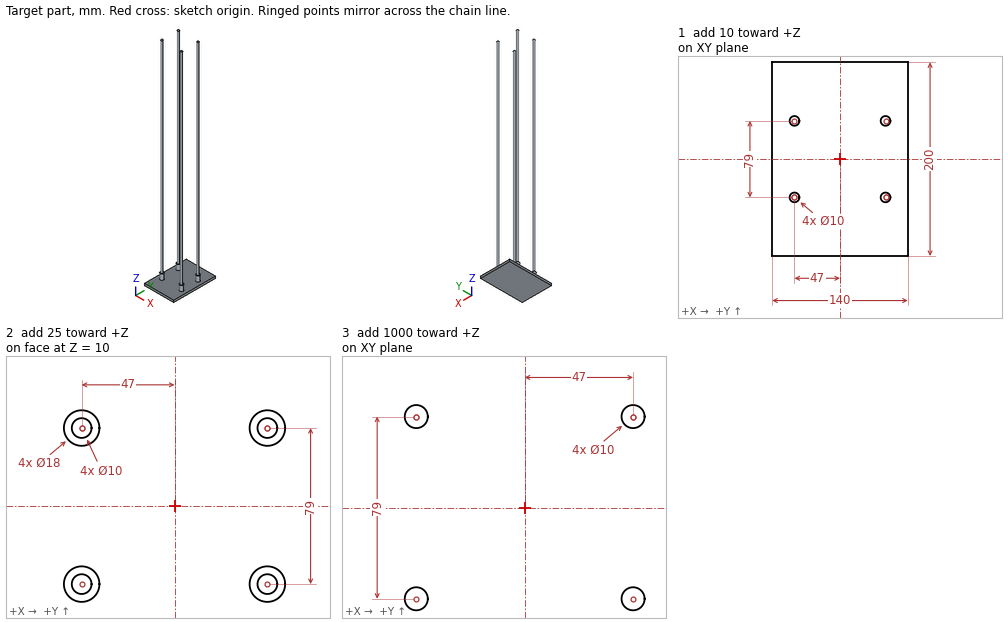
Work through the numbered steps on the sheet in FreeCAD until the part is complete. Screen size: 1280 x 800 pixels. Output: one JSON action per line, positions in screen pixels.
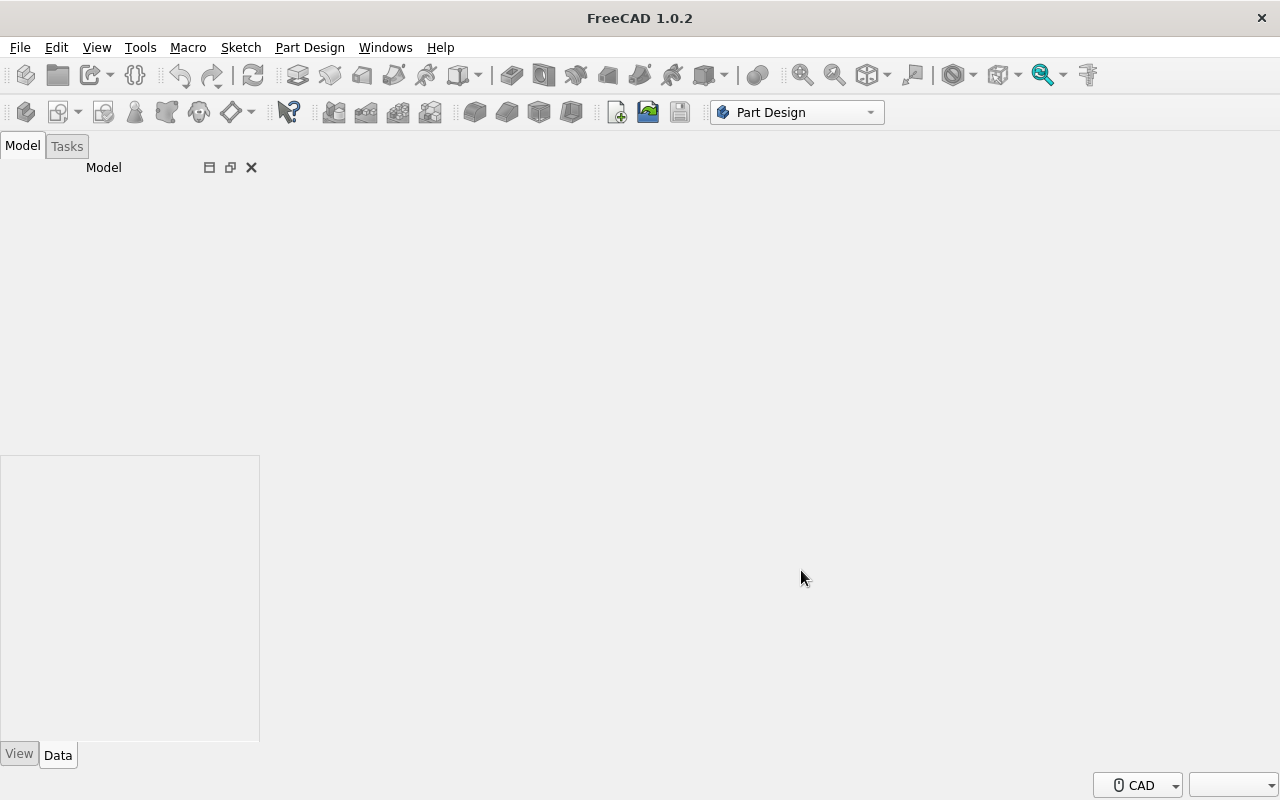
{"action": "left_click", "coordinate": [616, 112]}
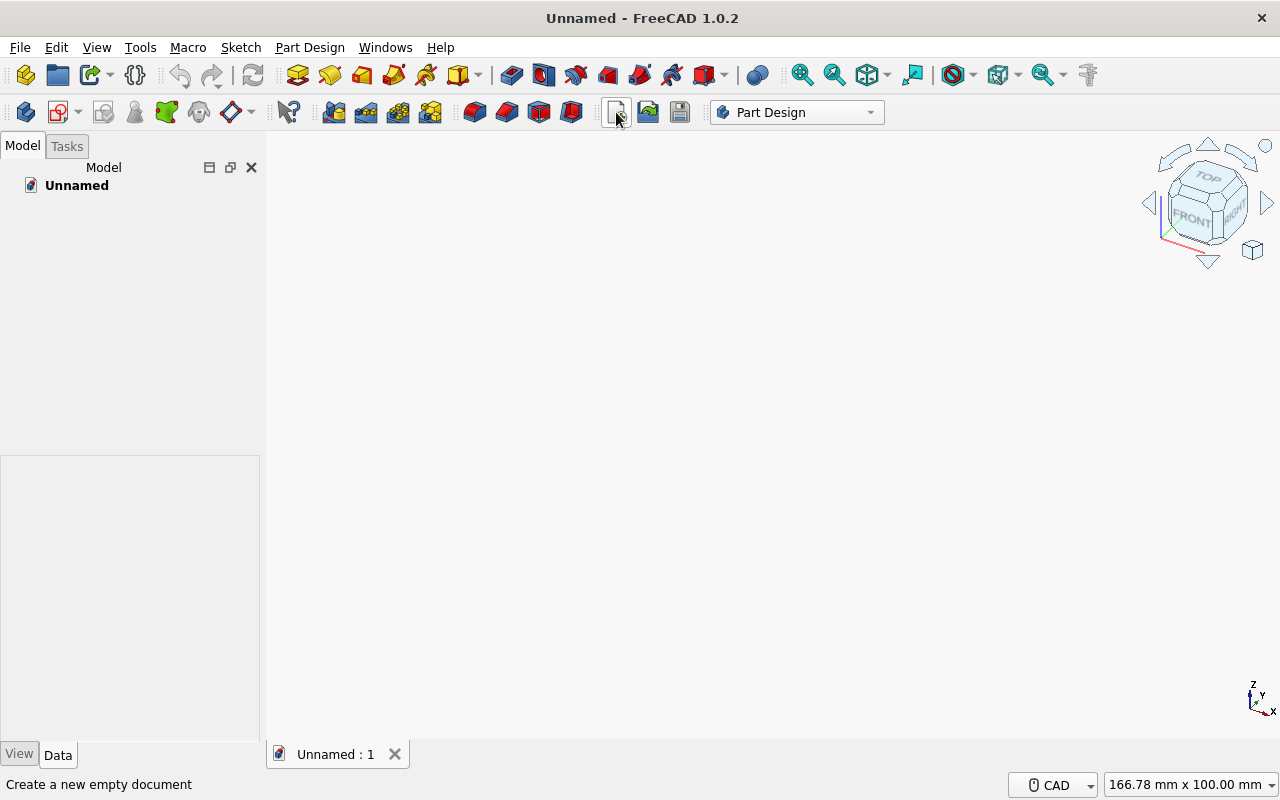
{"action": "left_click", "coordinate": [58, 112]}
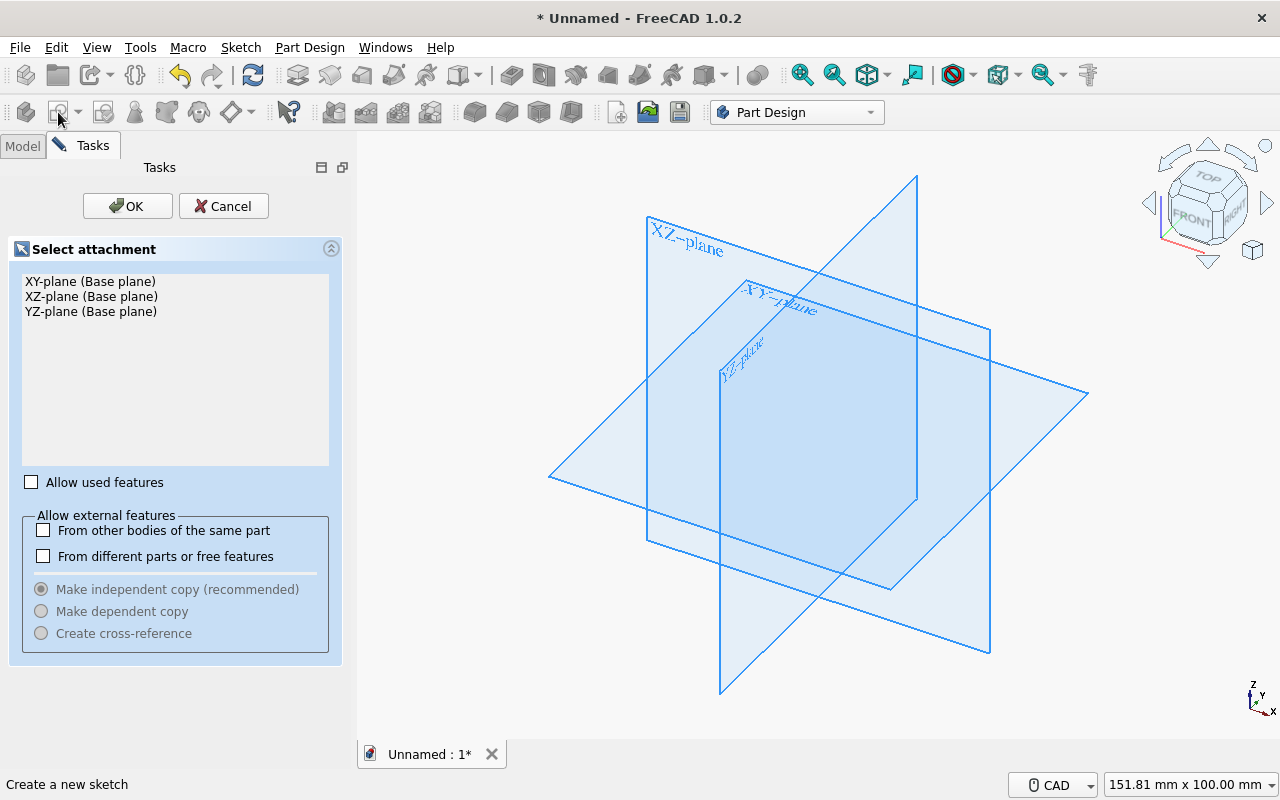
{"action": "left_click", "coordinate": [82, 282]}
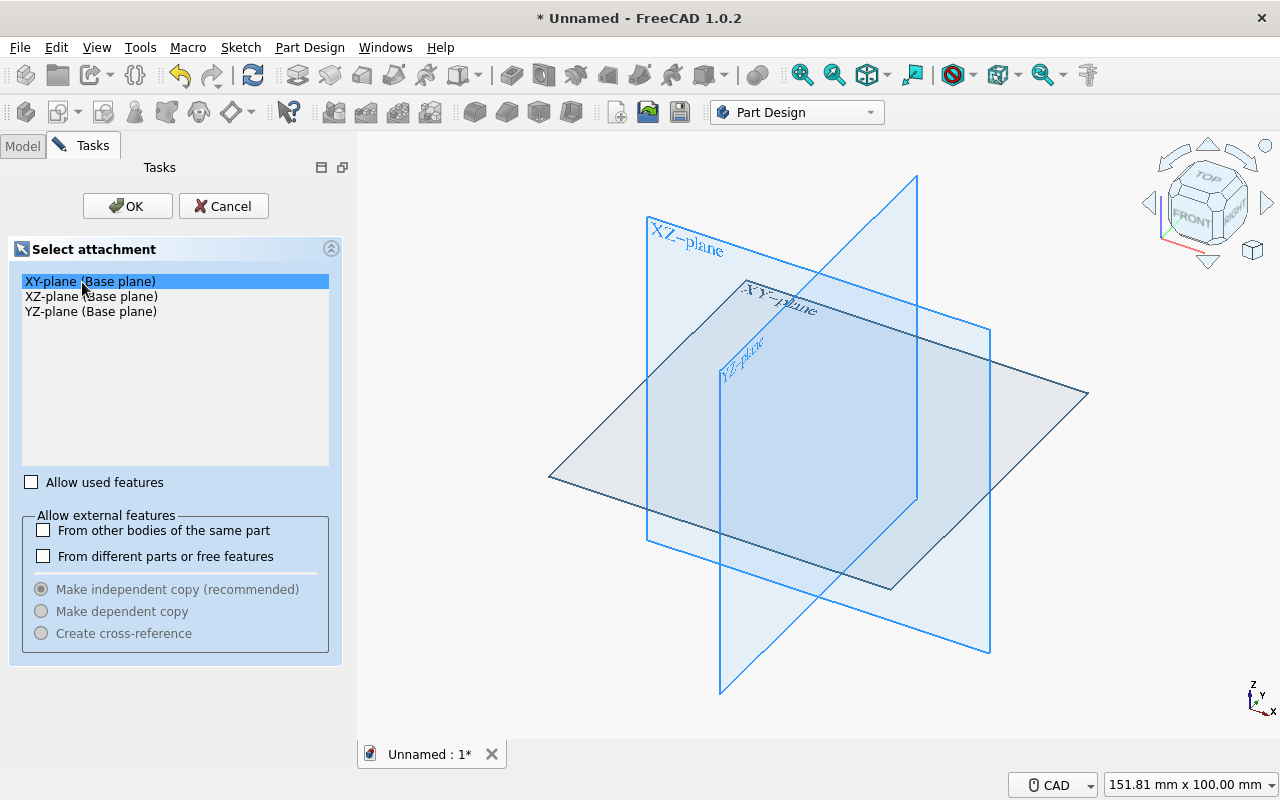
{"action": "left_click", "coordinate": [128, 206]}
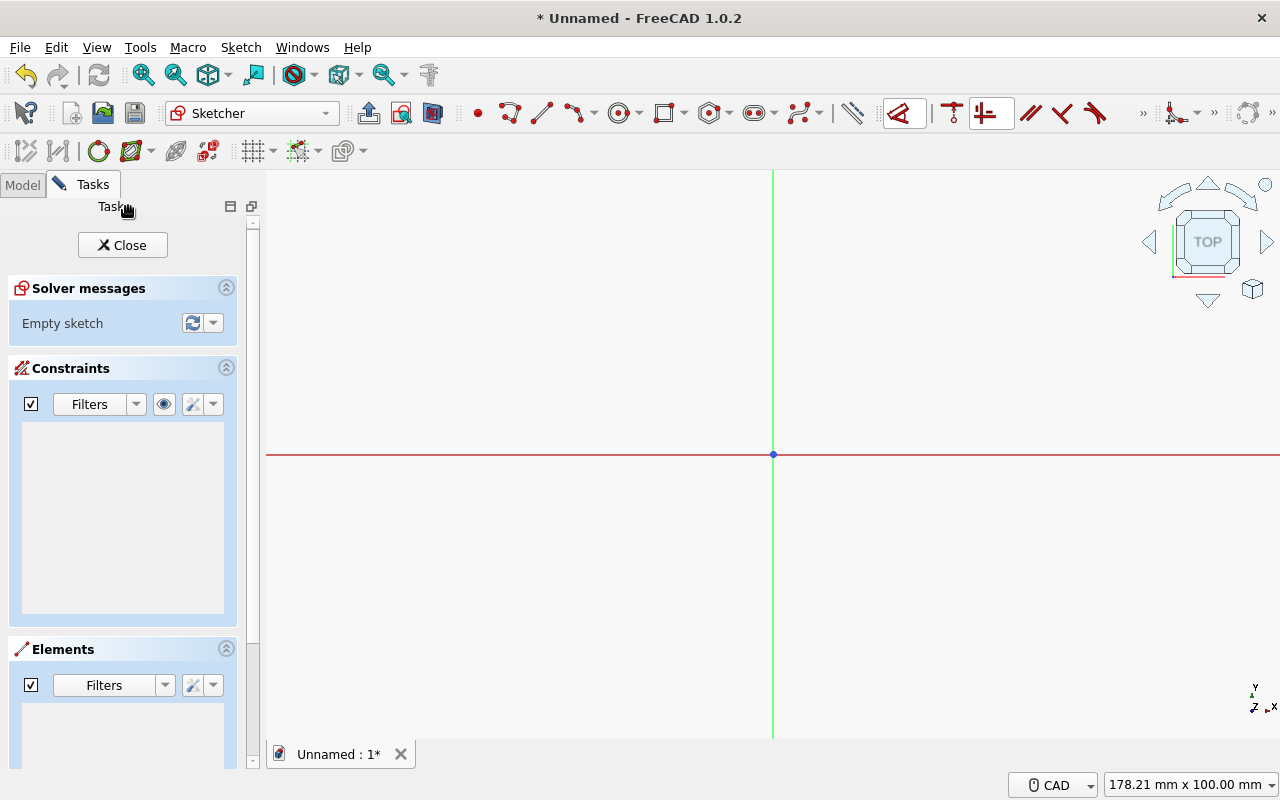
{"action": "scroll", "coordinate": [675, 454], "scroll_direction": "down", "scroll_amount": 6}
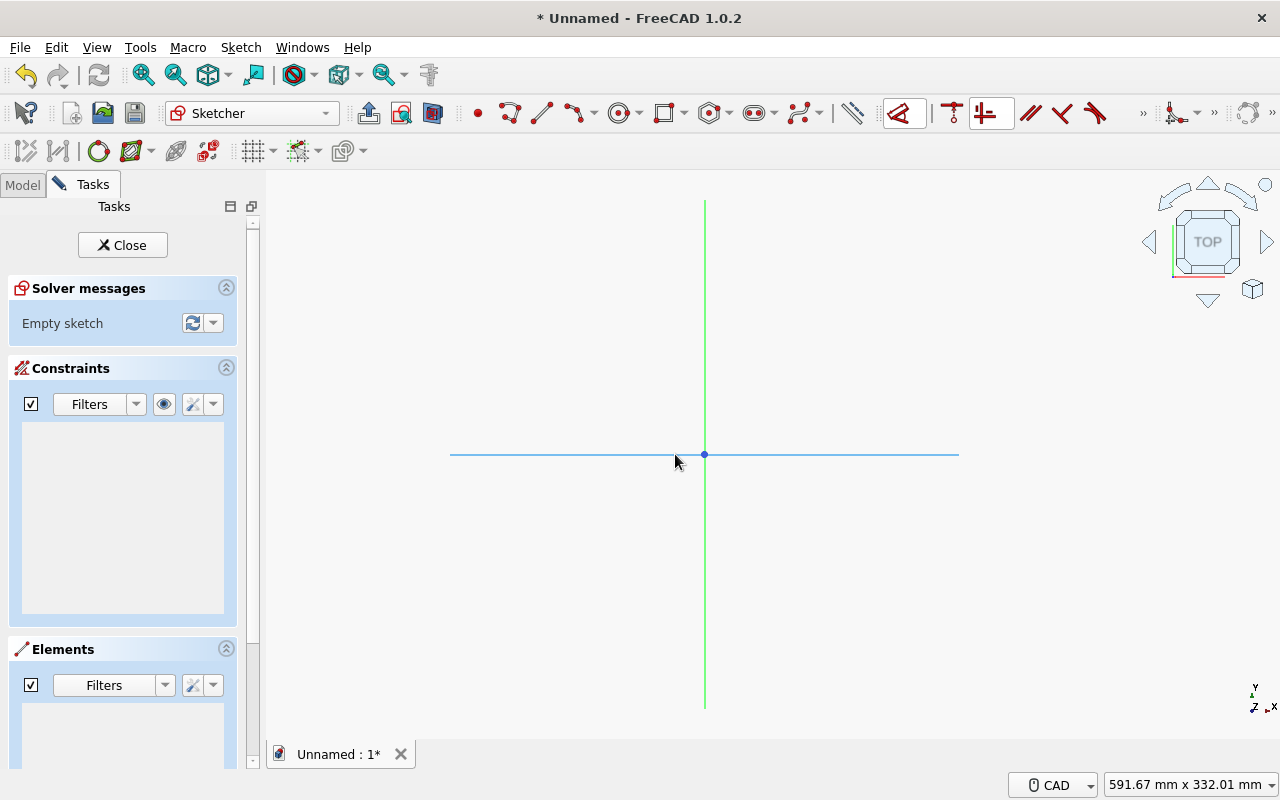
{"action": "left_click", "coordinate": [686, 114]}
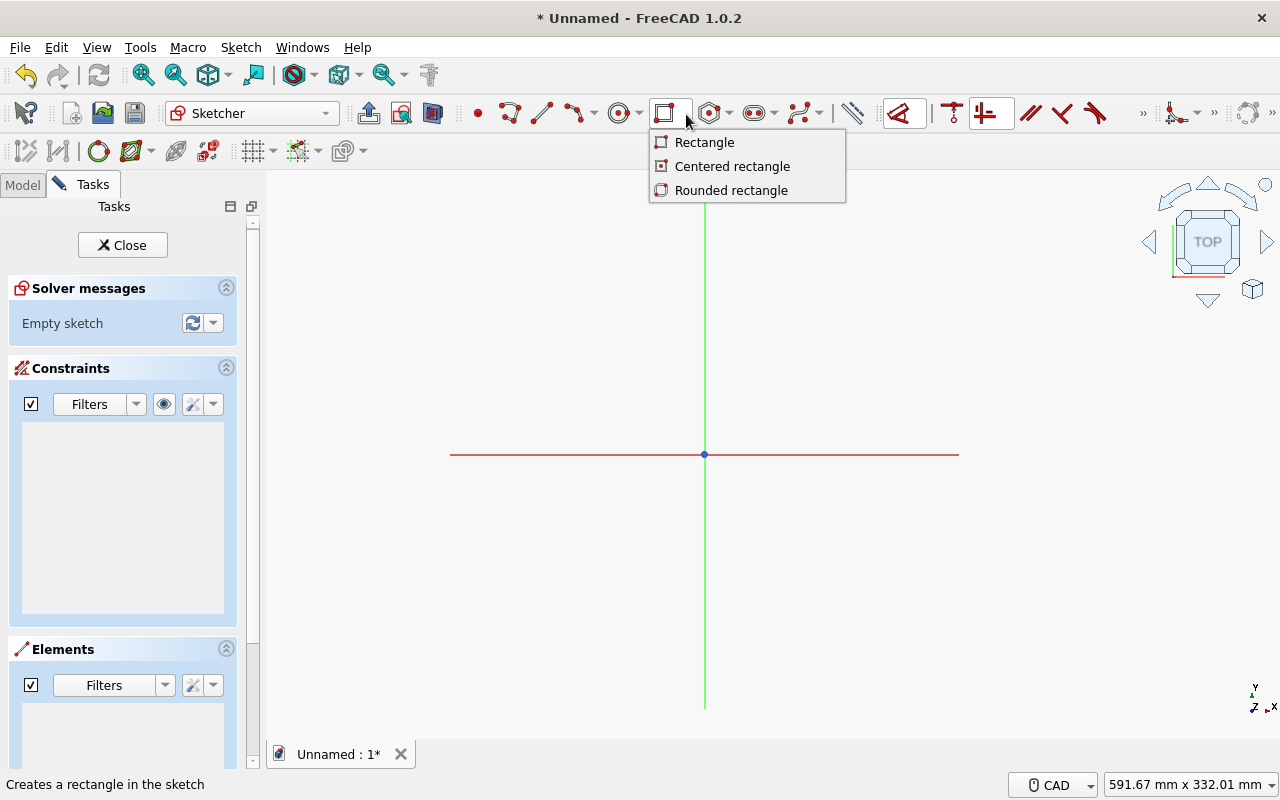
{"action": "left_click", "coordinate": [748, 166]}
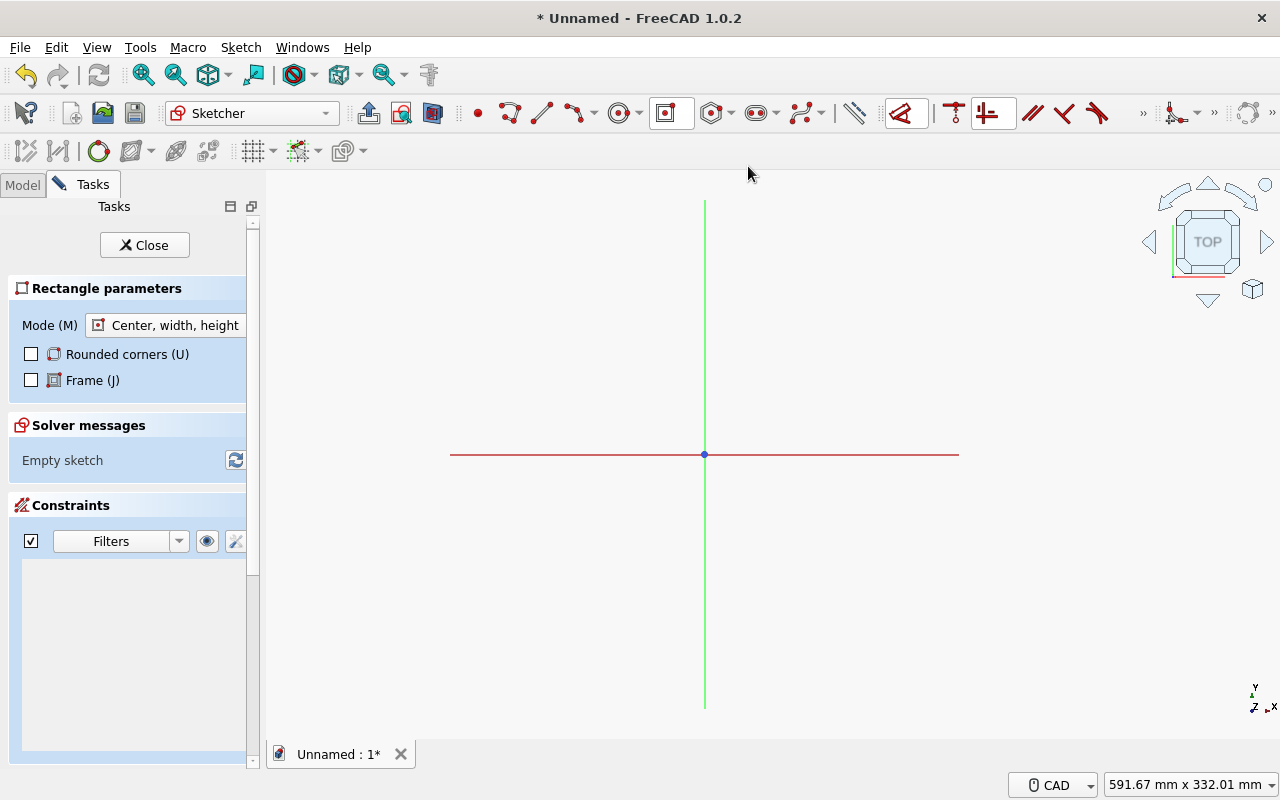
{"action": "left_click", "coordinate": [705, 454]}
{"action": "left_click", "coordinate": [825, 283]}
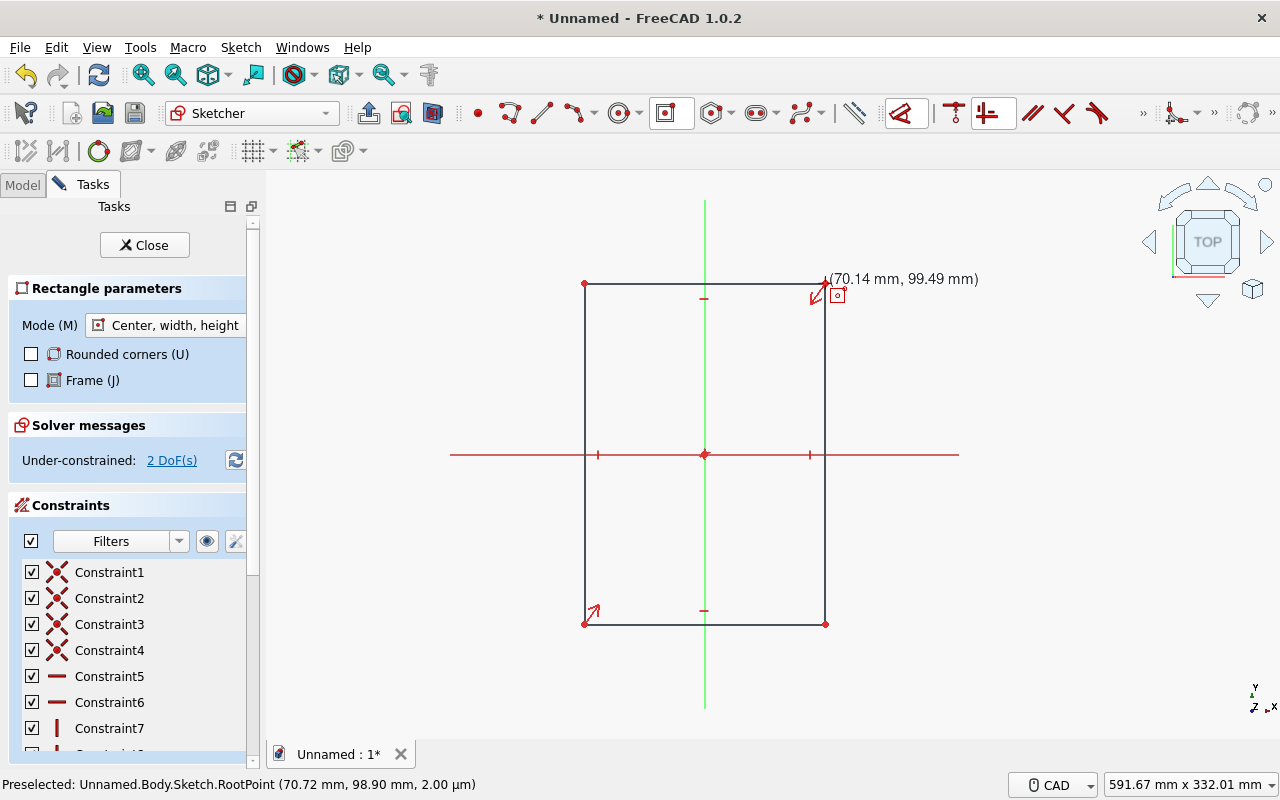
{"action": "left_click", "coordinate": [620, 114]}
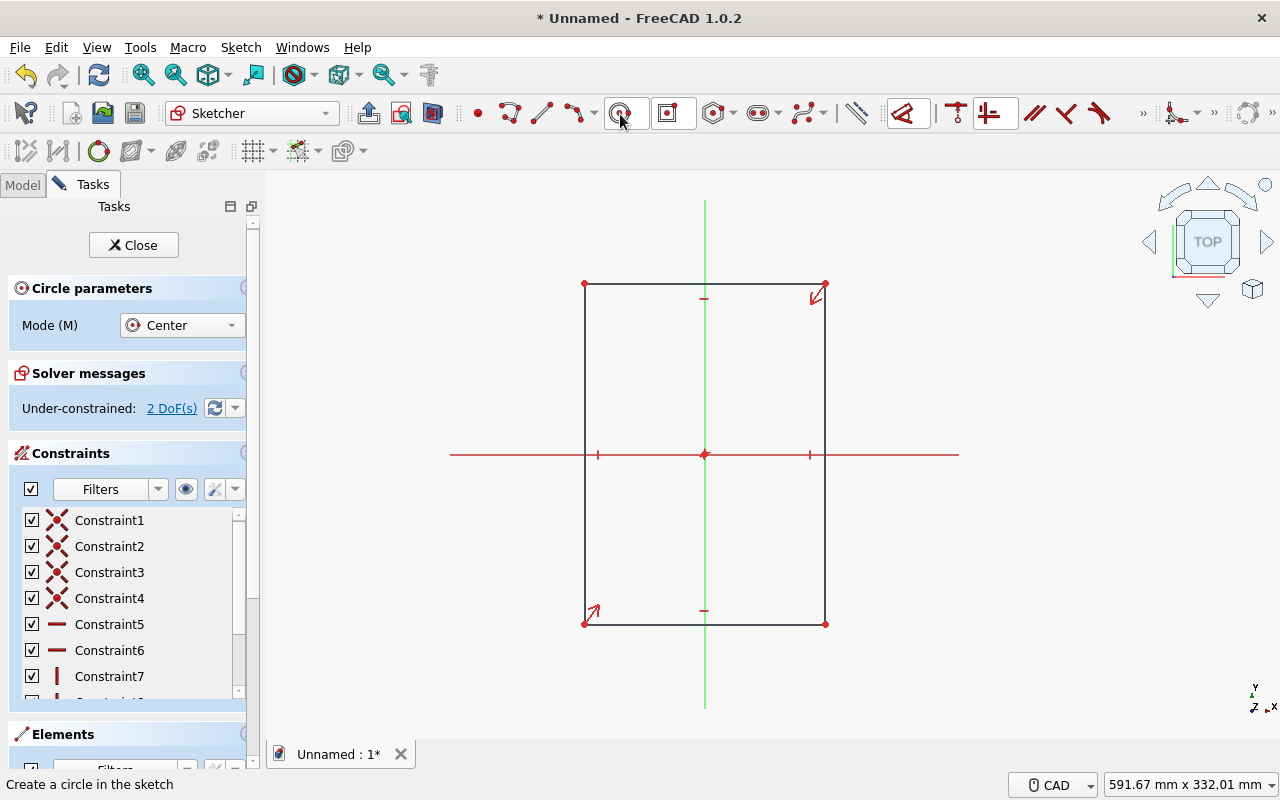
{"action": "scroll", "coordinate": [624, 522], "scroll_direction": "up", "scroll_amount": 5}